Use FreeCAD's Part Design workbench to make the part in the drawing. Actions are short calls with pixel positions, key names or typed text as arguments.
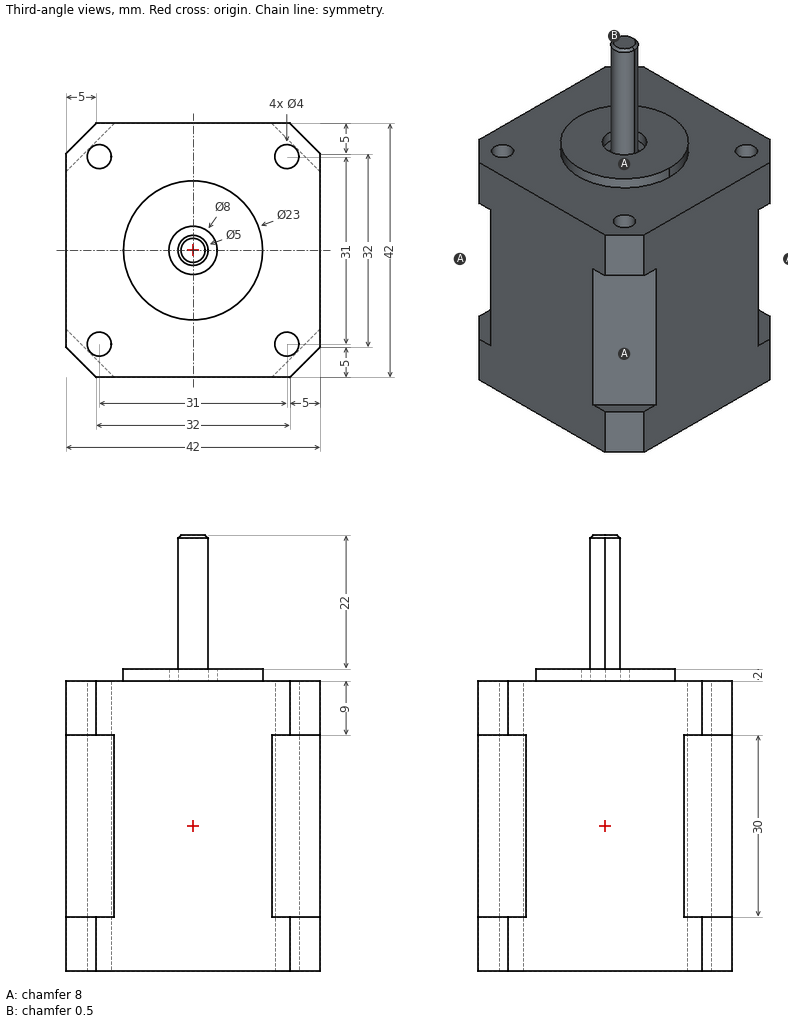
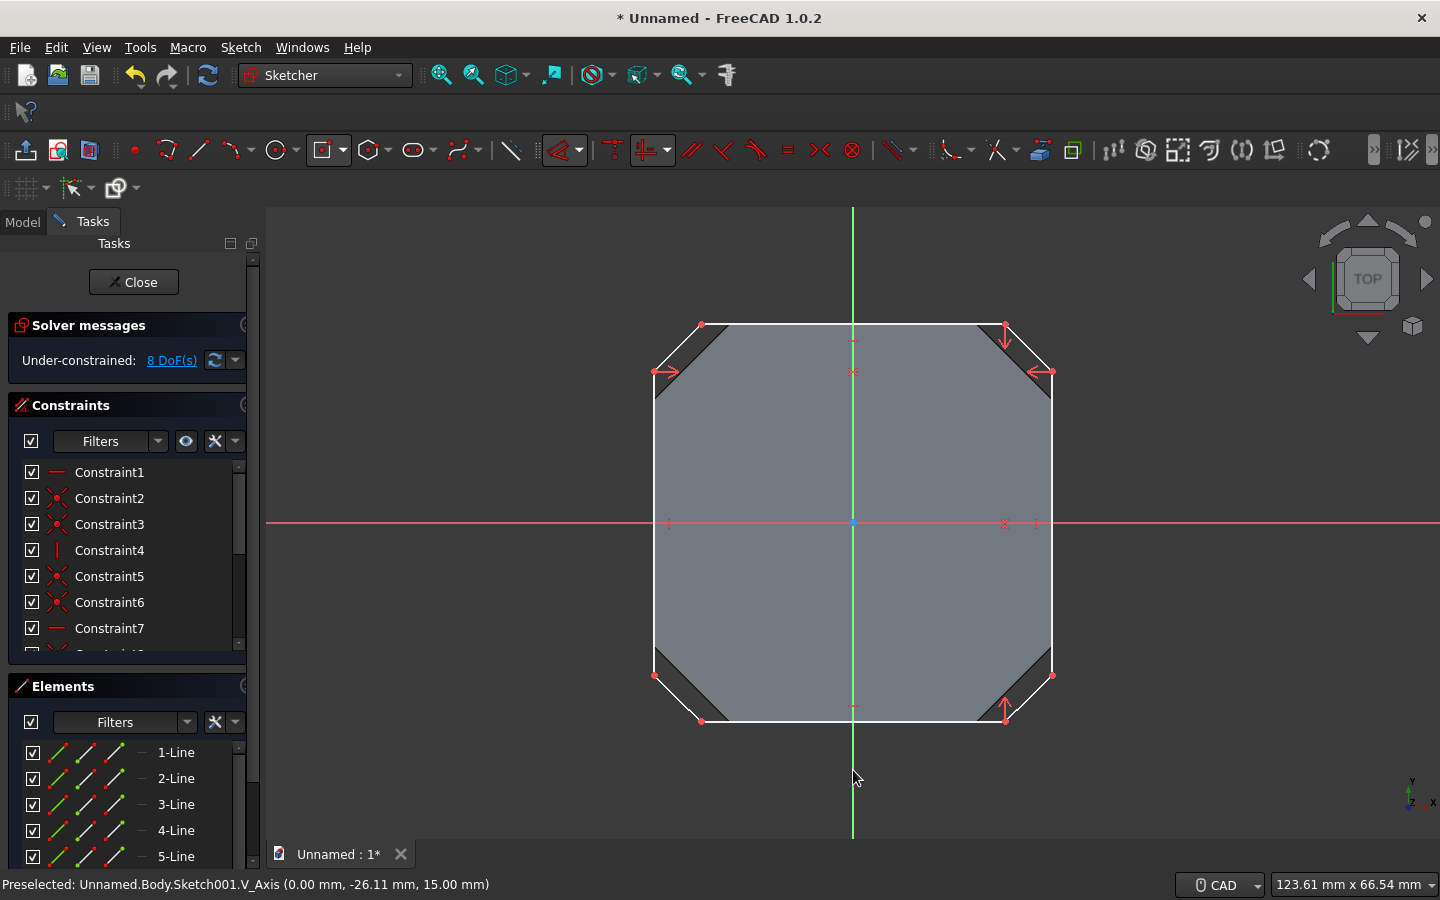
click(792, 722)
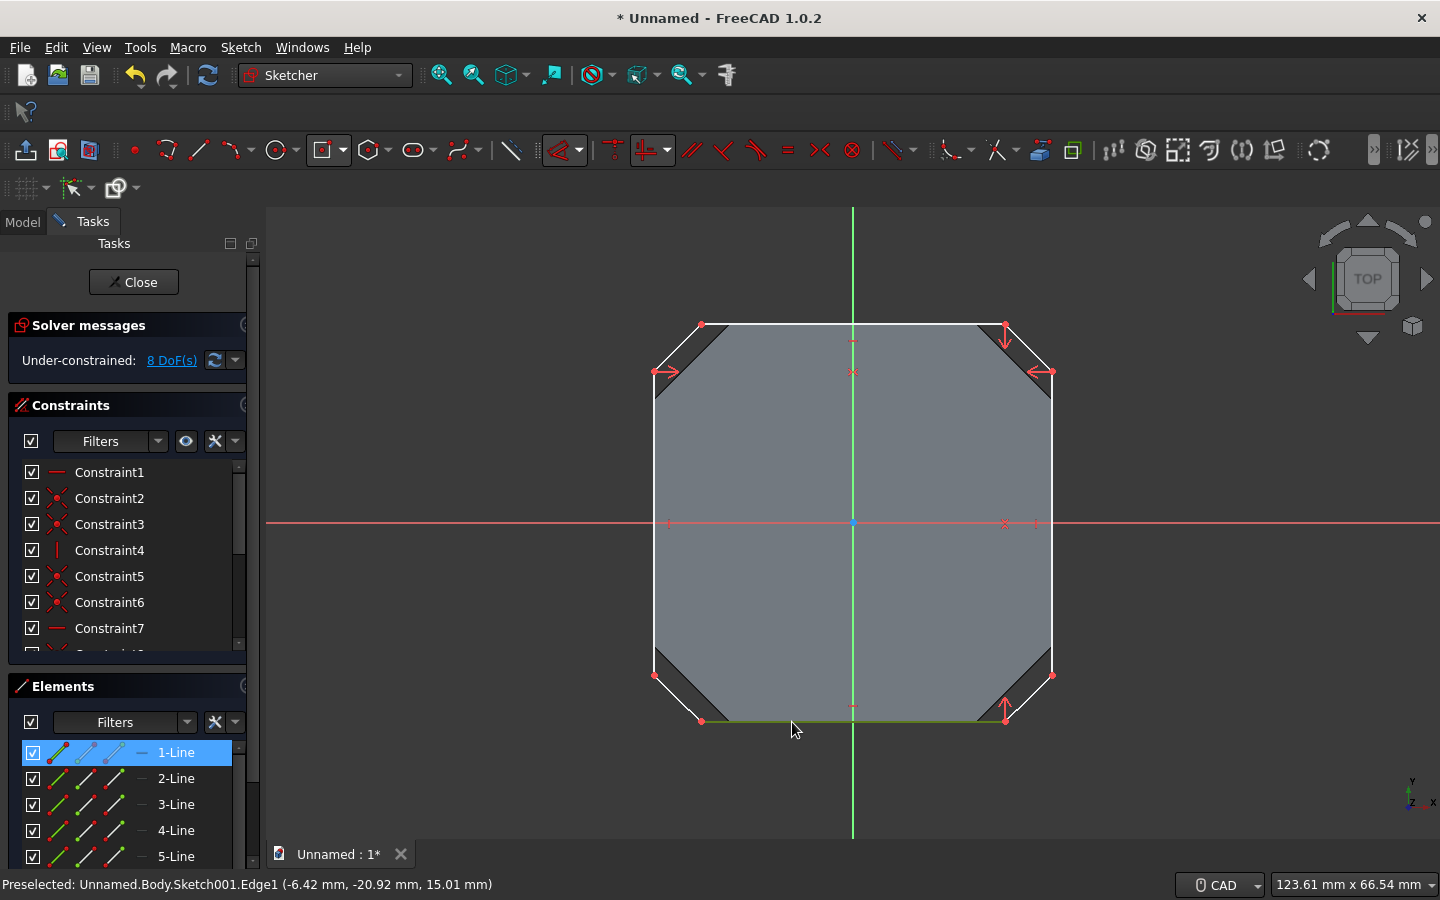
click(582, 150)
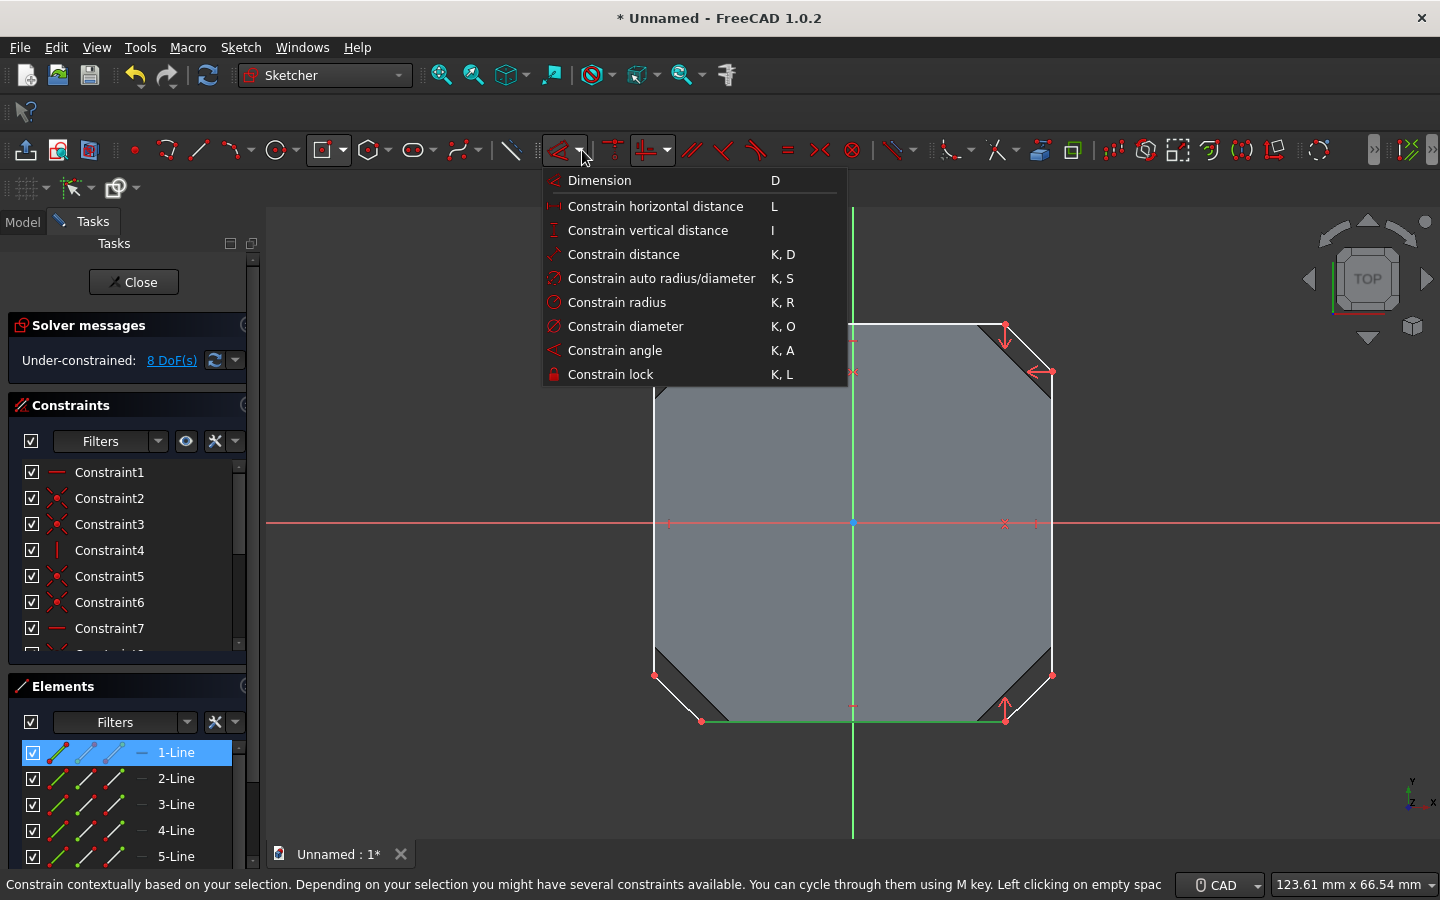
click(695, 206)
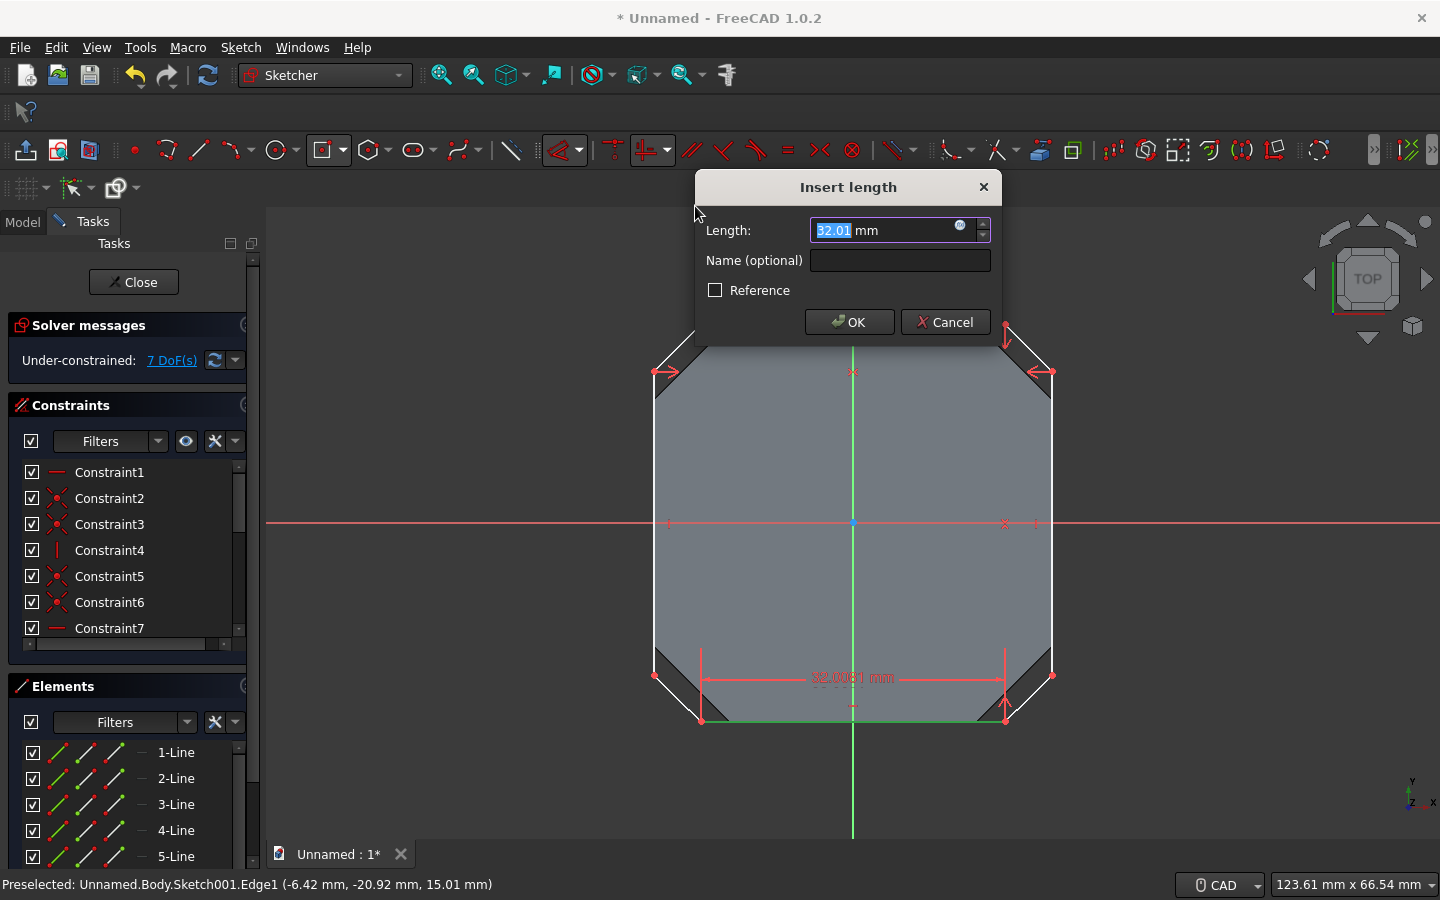
text(32)
key(Return)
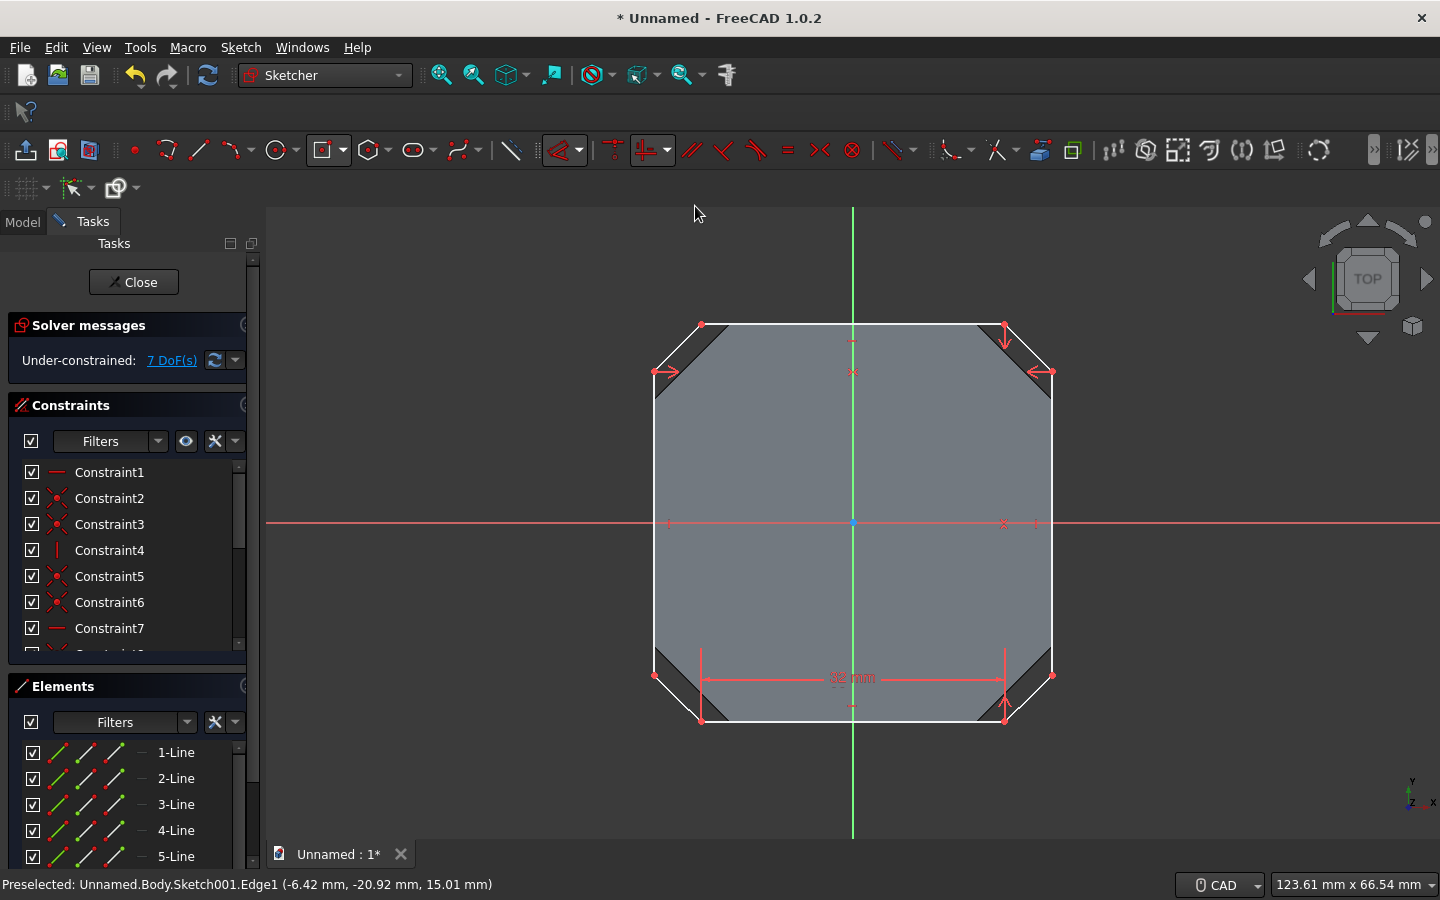
click(1052, 585)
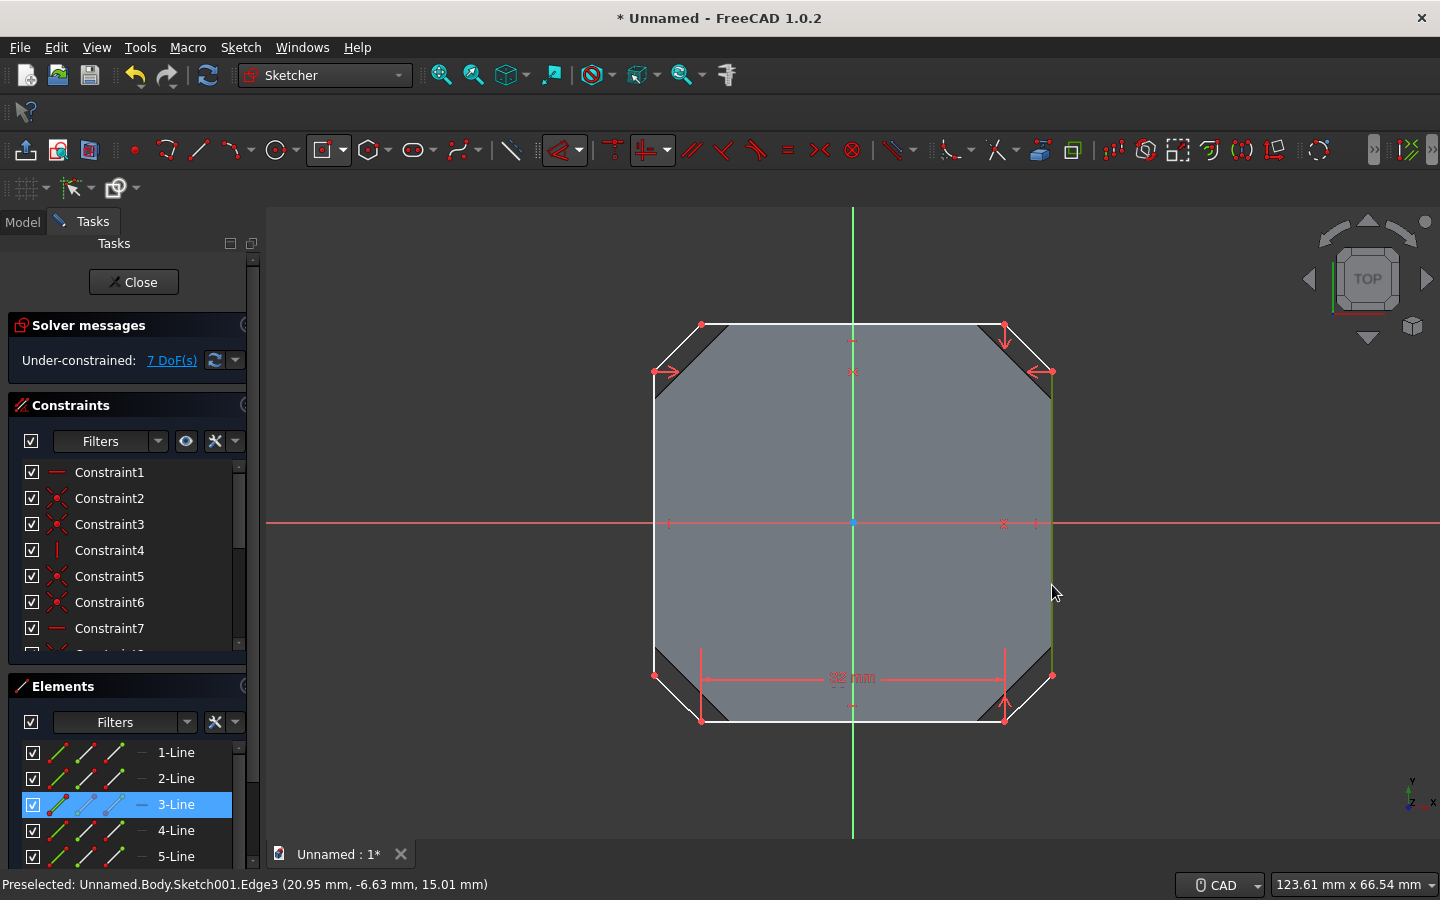
click(582, 150)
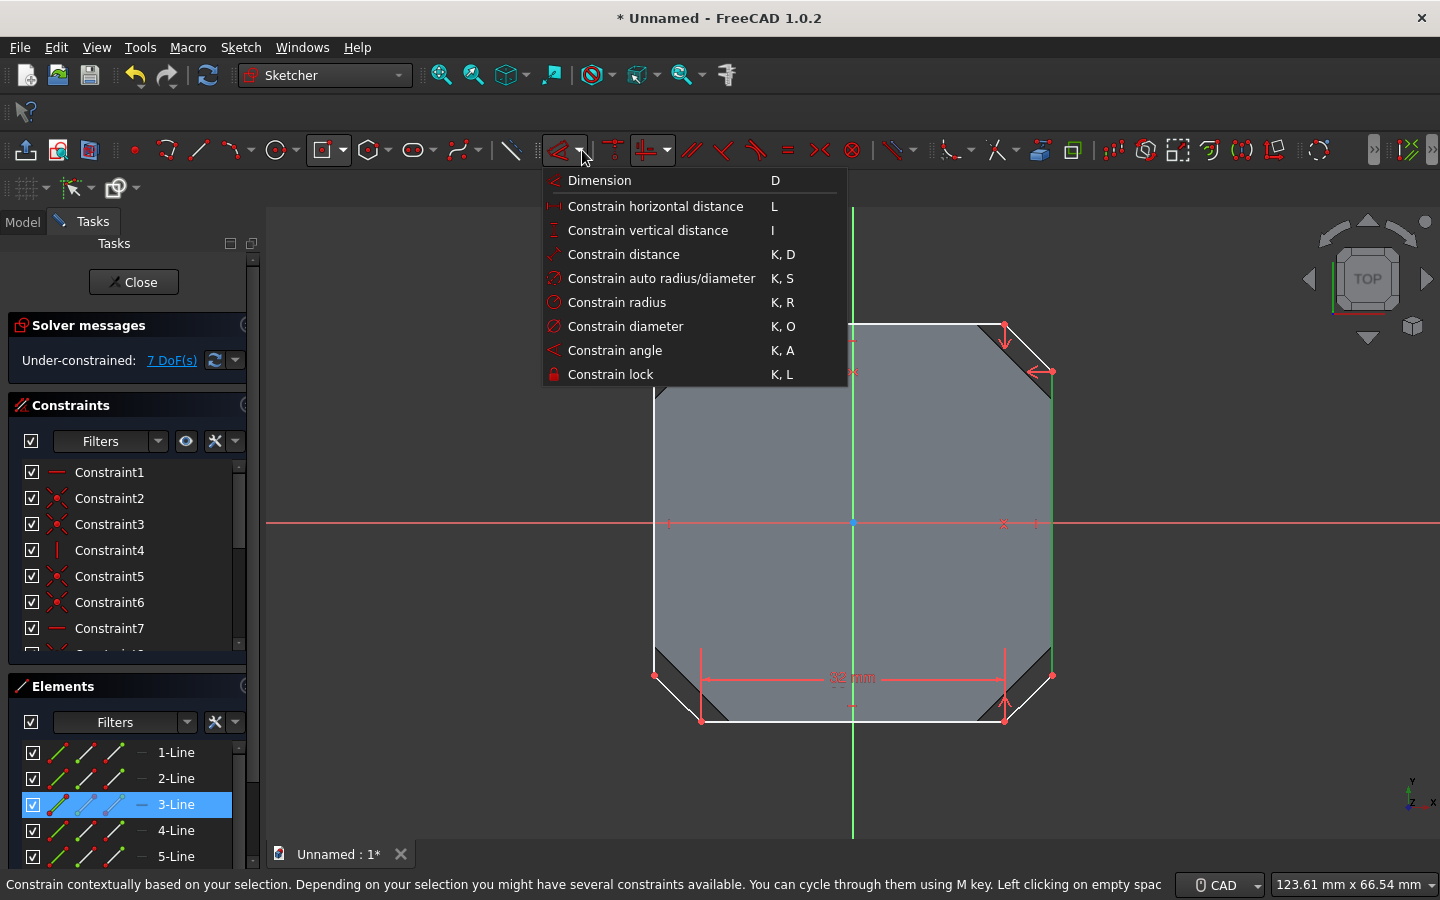
click(695, 230)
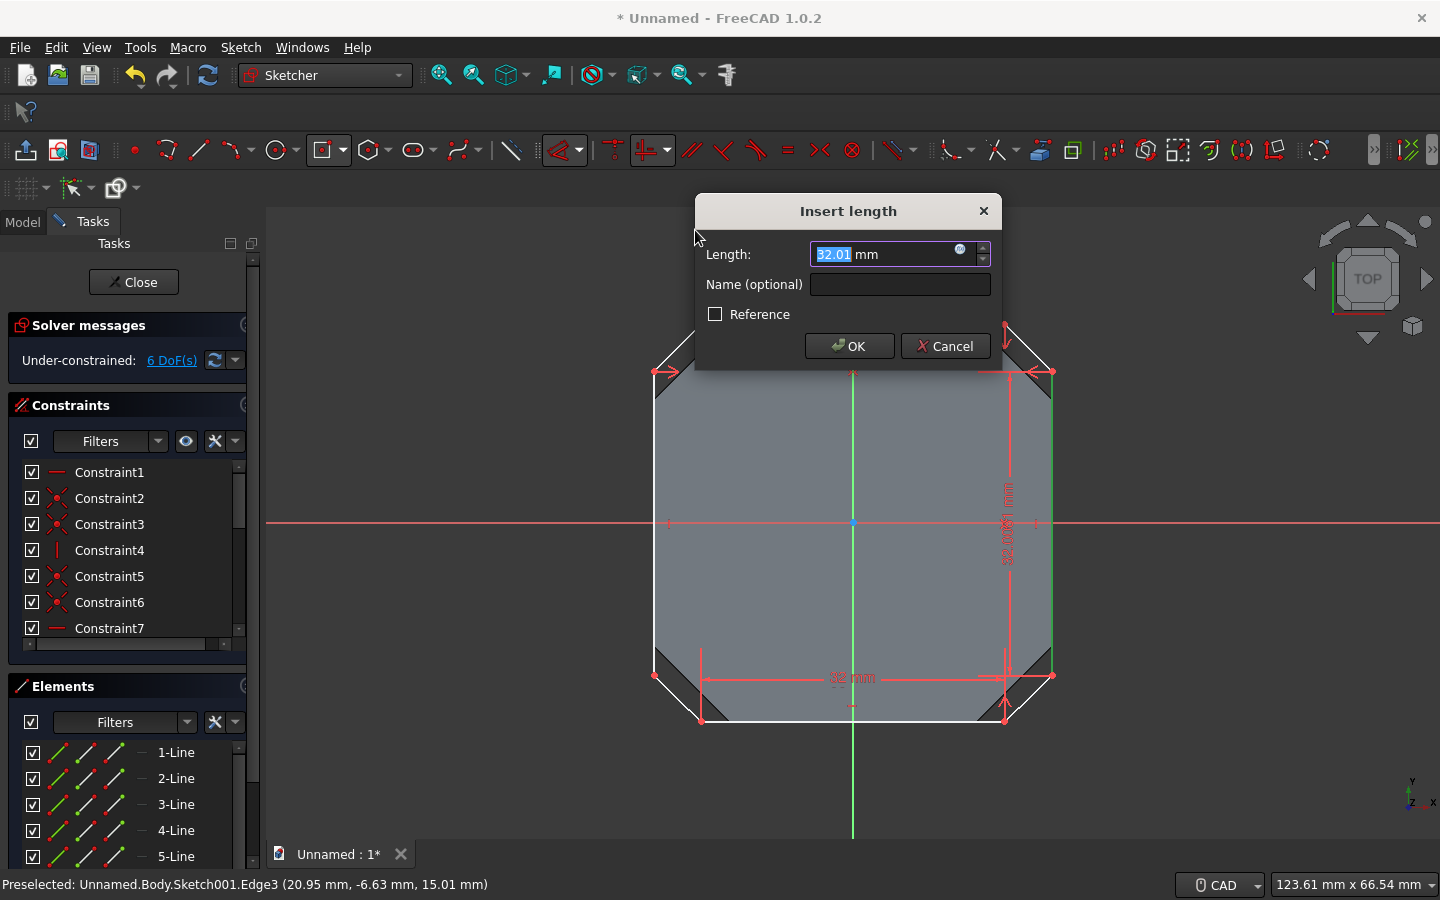
text(32)
key(Return)